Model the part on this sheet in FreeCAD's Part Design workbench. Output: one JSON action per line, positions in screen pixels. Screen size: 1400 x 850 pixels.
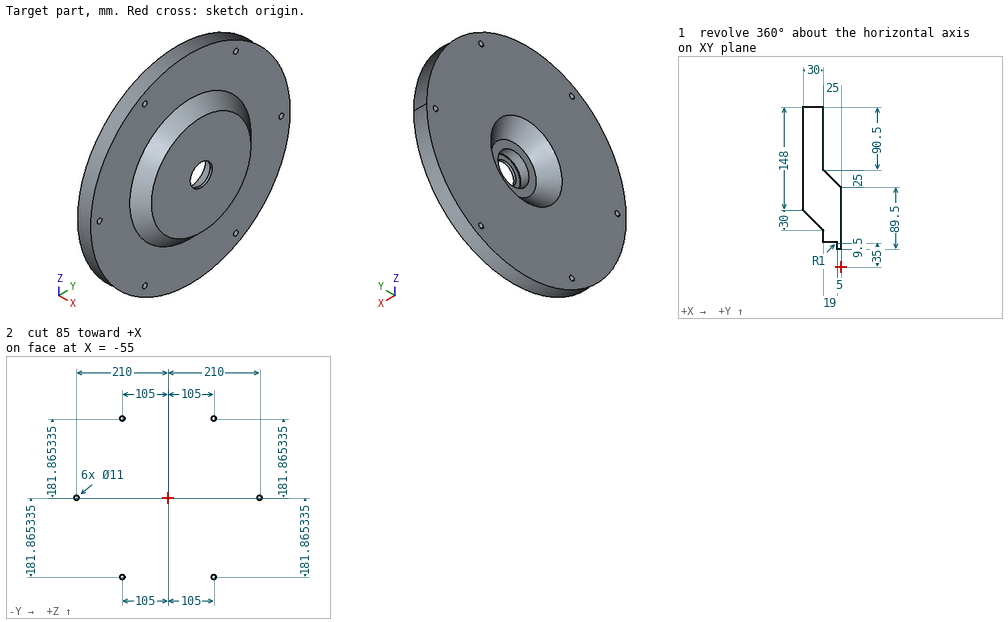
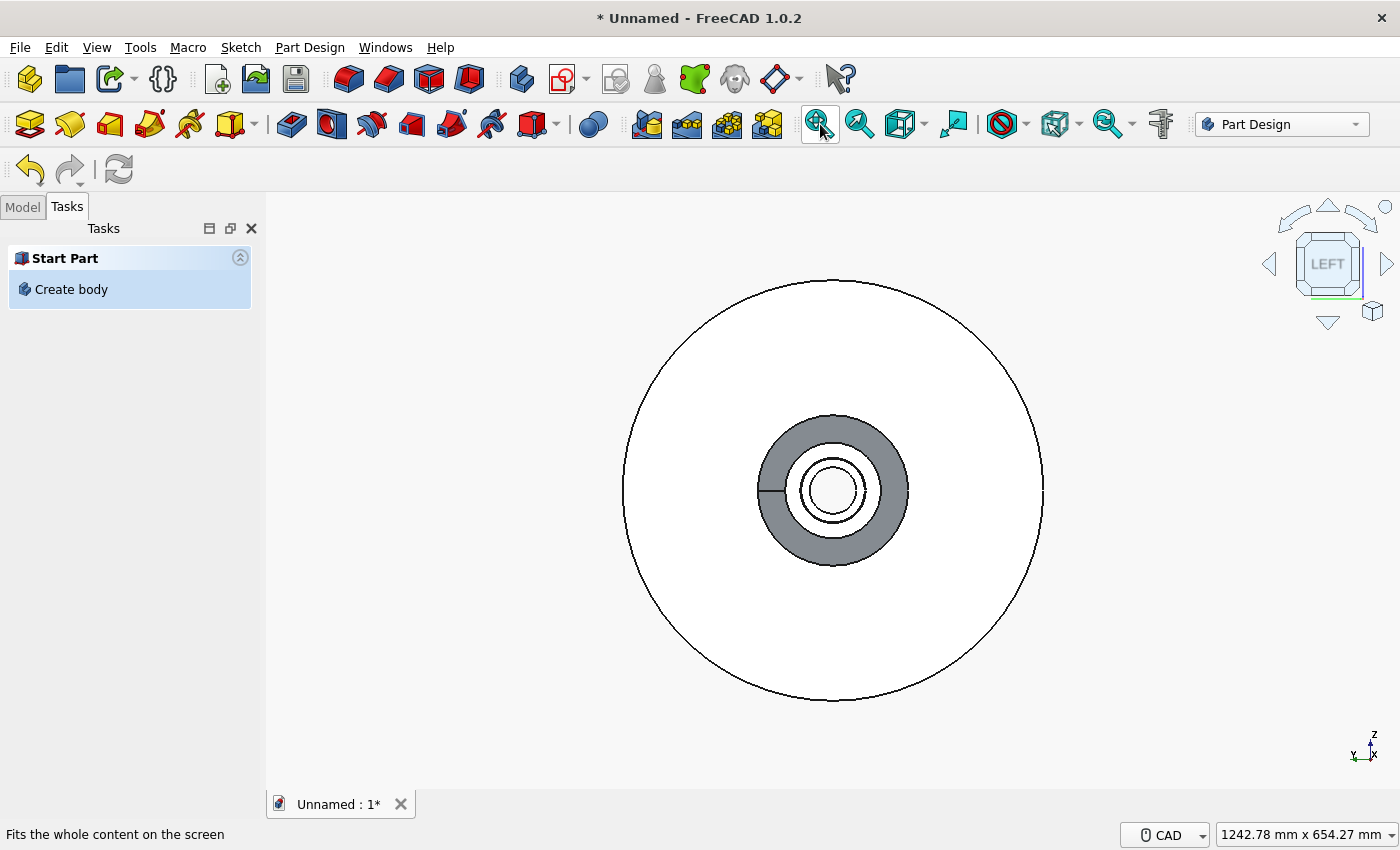
{"action": "left_click", "coordinate": [713, 550]}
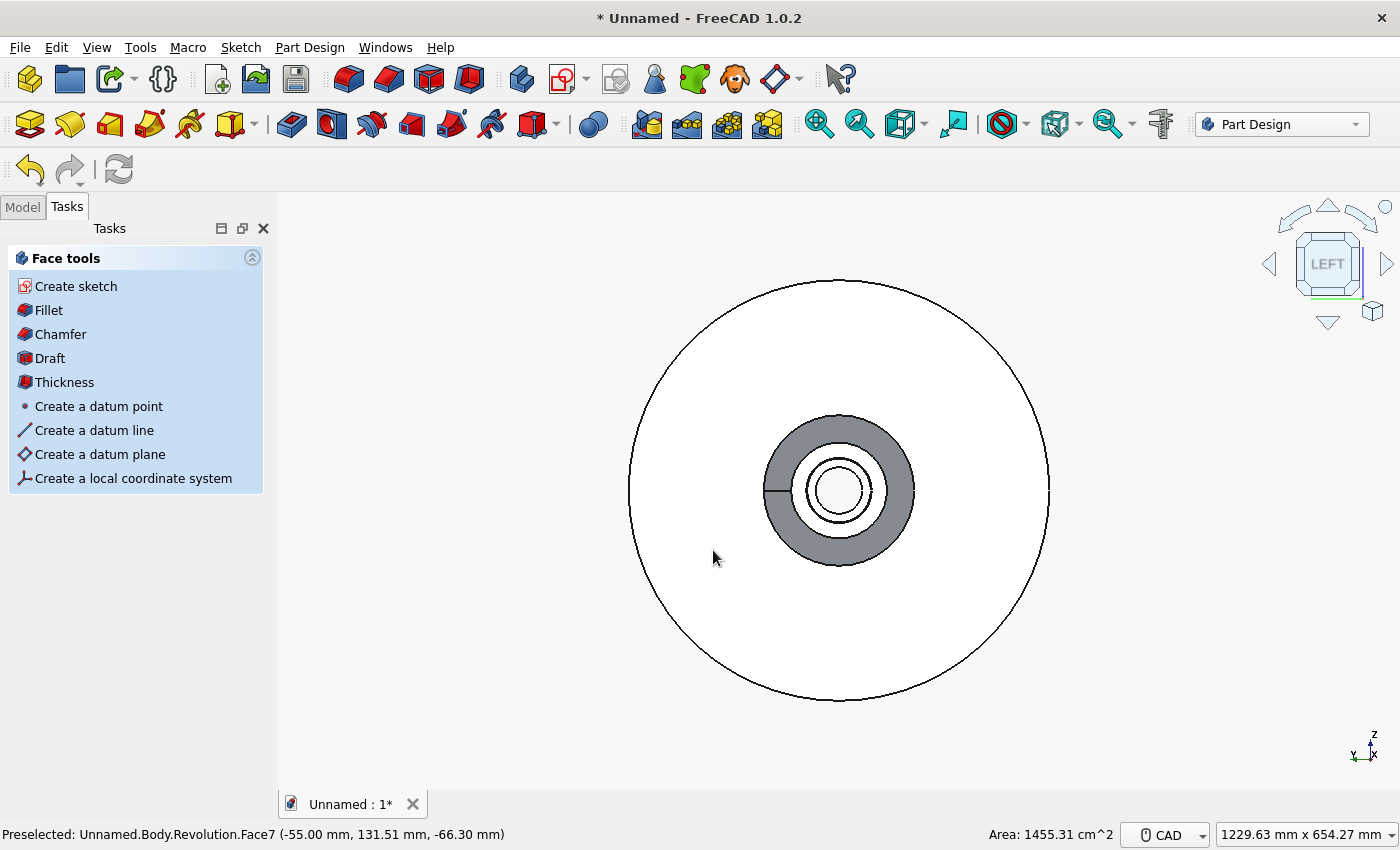
{"action": "left_click", "coordinate": [562, 80]}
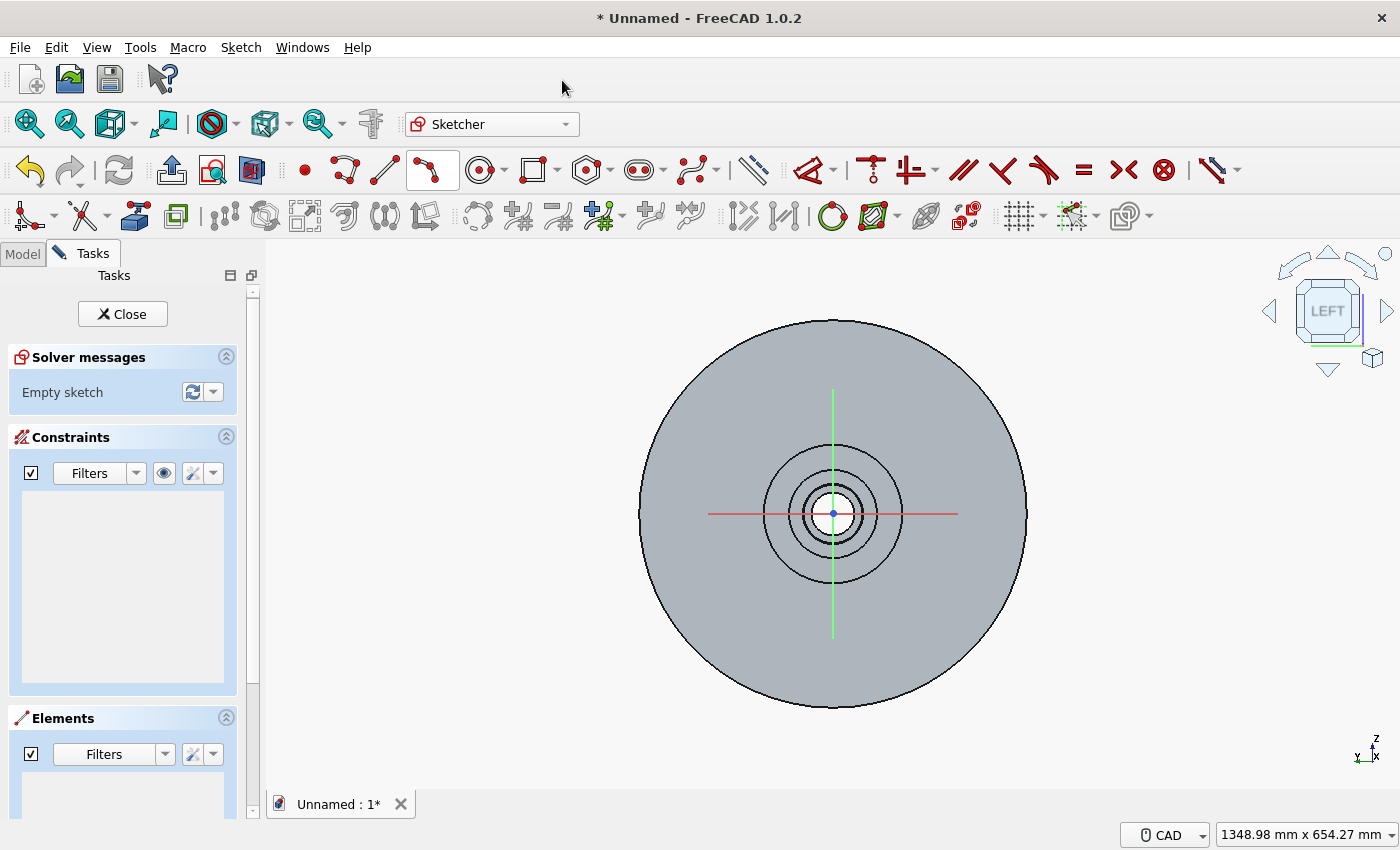
{"action": "left_click", "coordinate": [480, 170]}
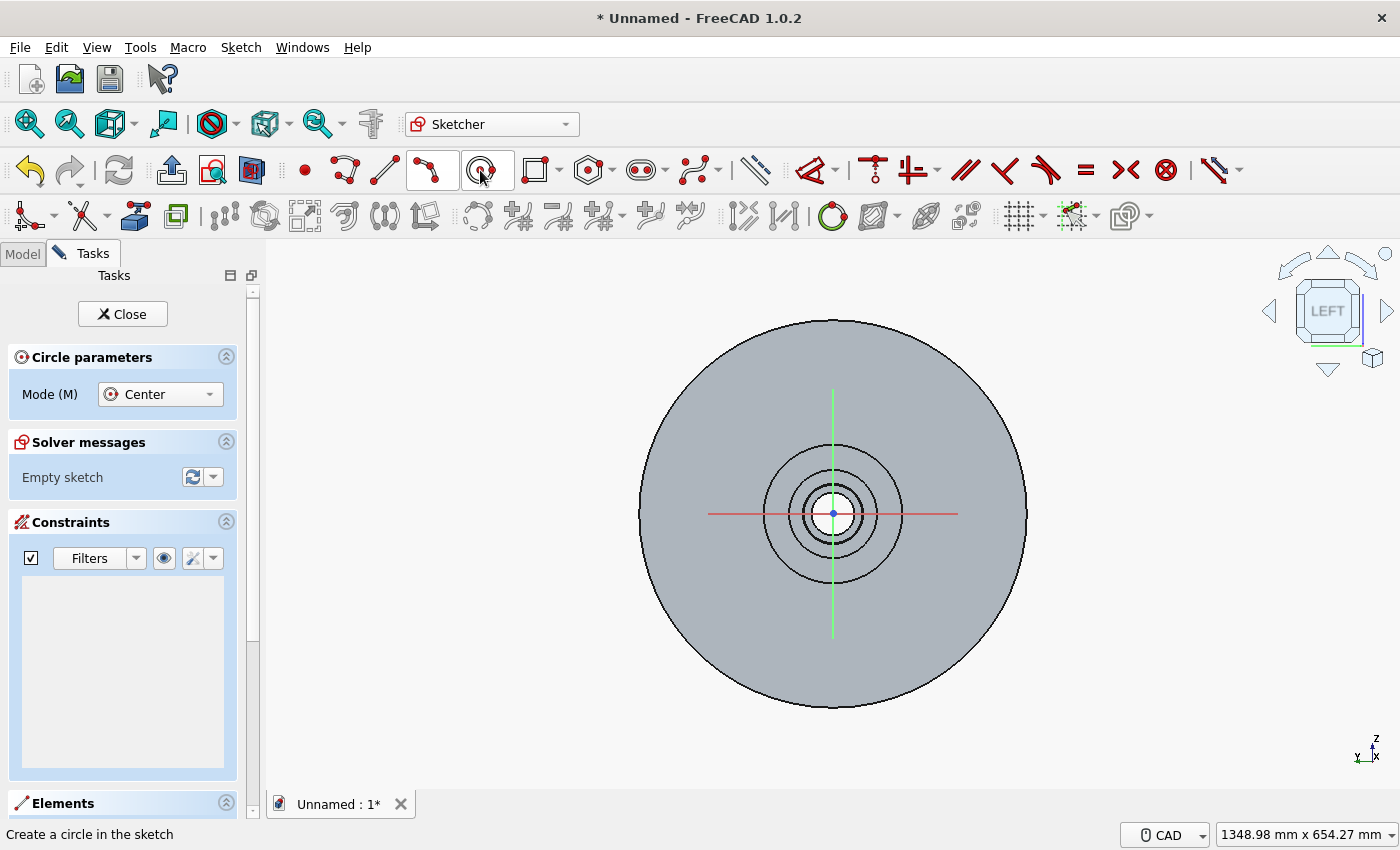
{"action": "scroll", "coordinate": [656, 514], "scroll_direction": "up", "scroll_amount": 8}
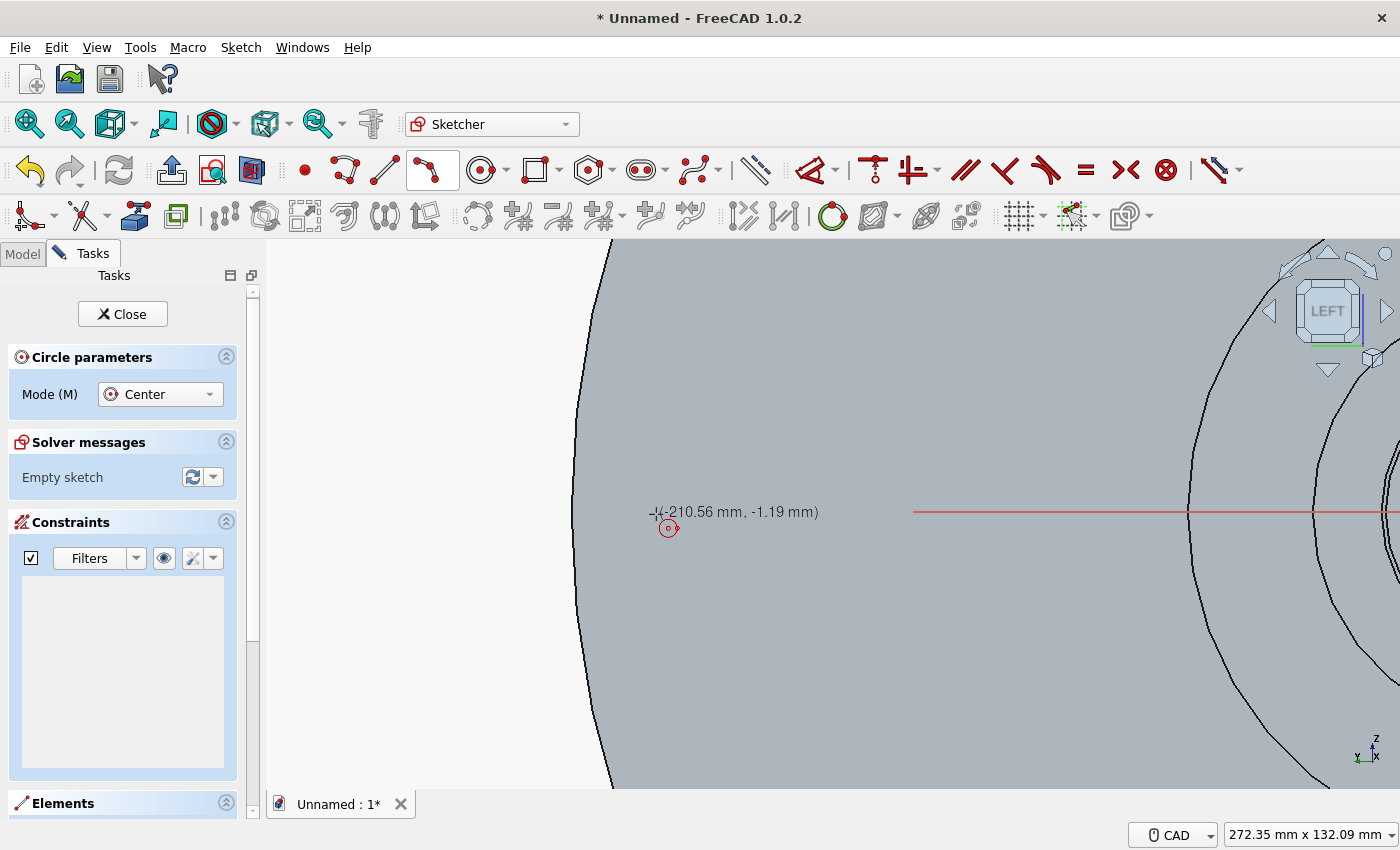
{"action": "scroll", "coordinate": [514, 515], "scroll_direction": "down", "scroll_amount": 7}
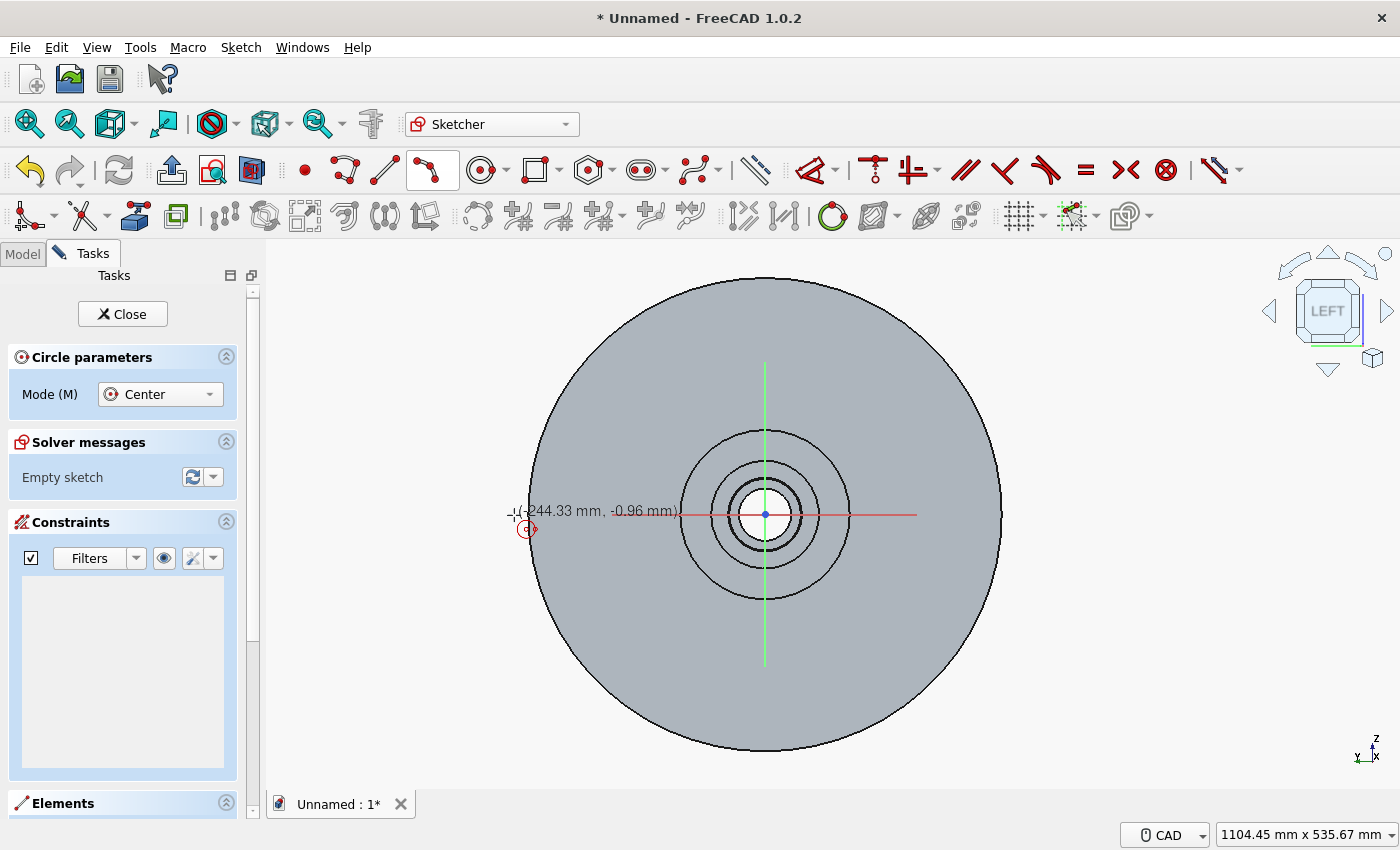
{"action": "left_click", "coordinate": [549, 515]}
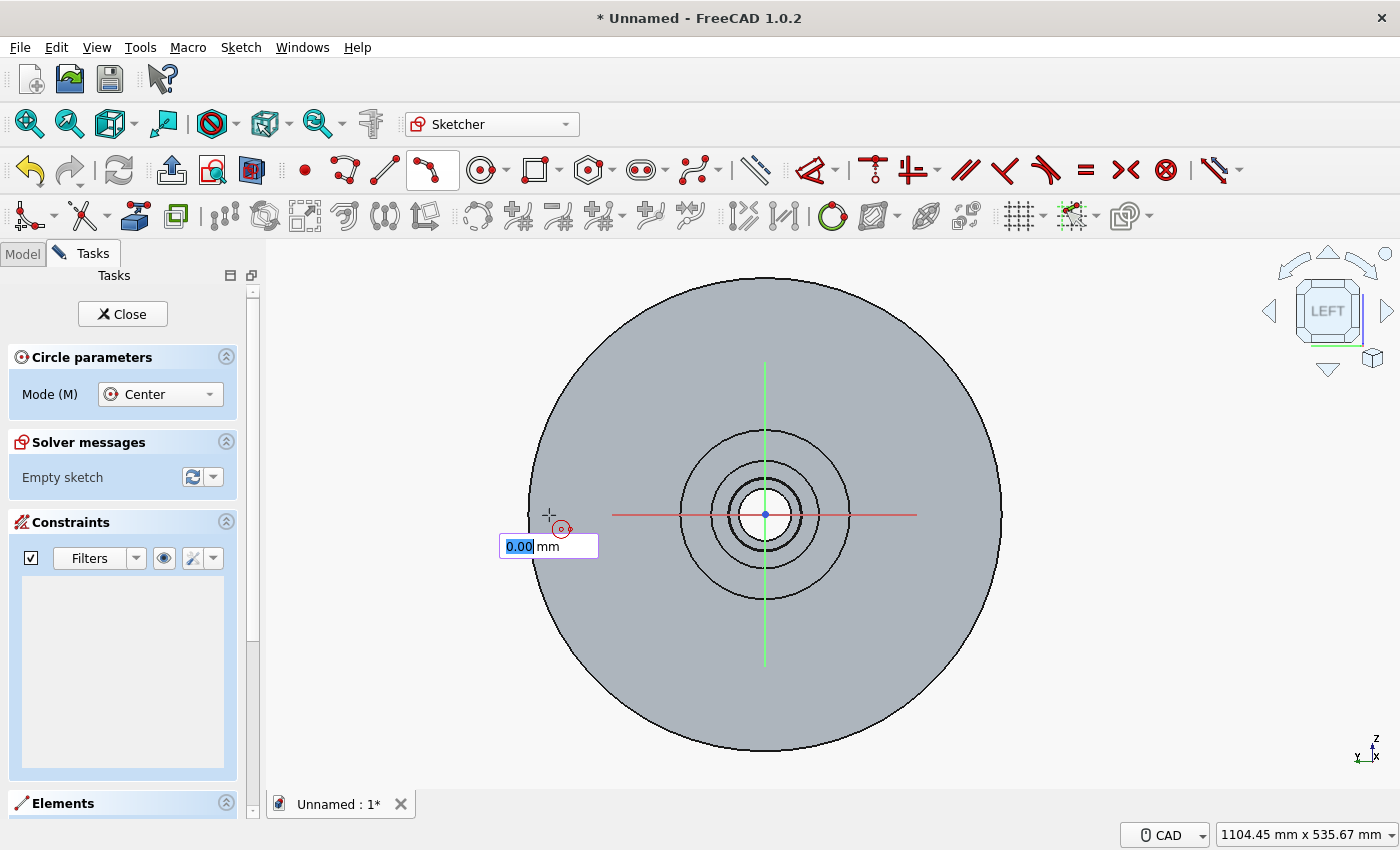
{"action": "scroll", "coordinate": [551, 509], "scroll_direction": "up", "scroll_amount": 6}
{"action": "mouse_move", "coordinate": [552, 509]}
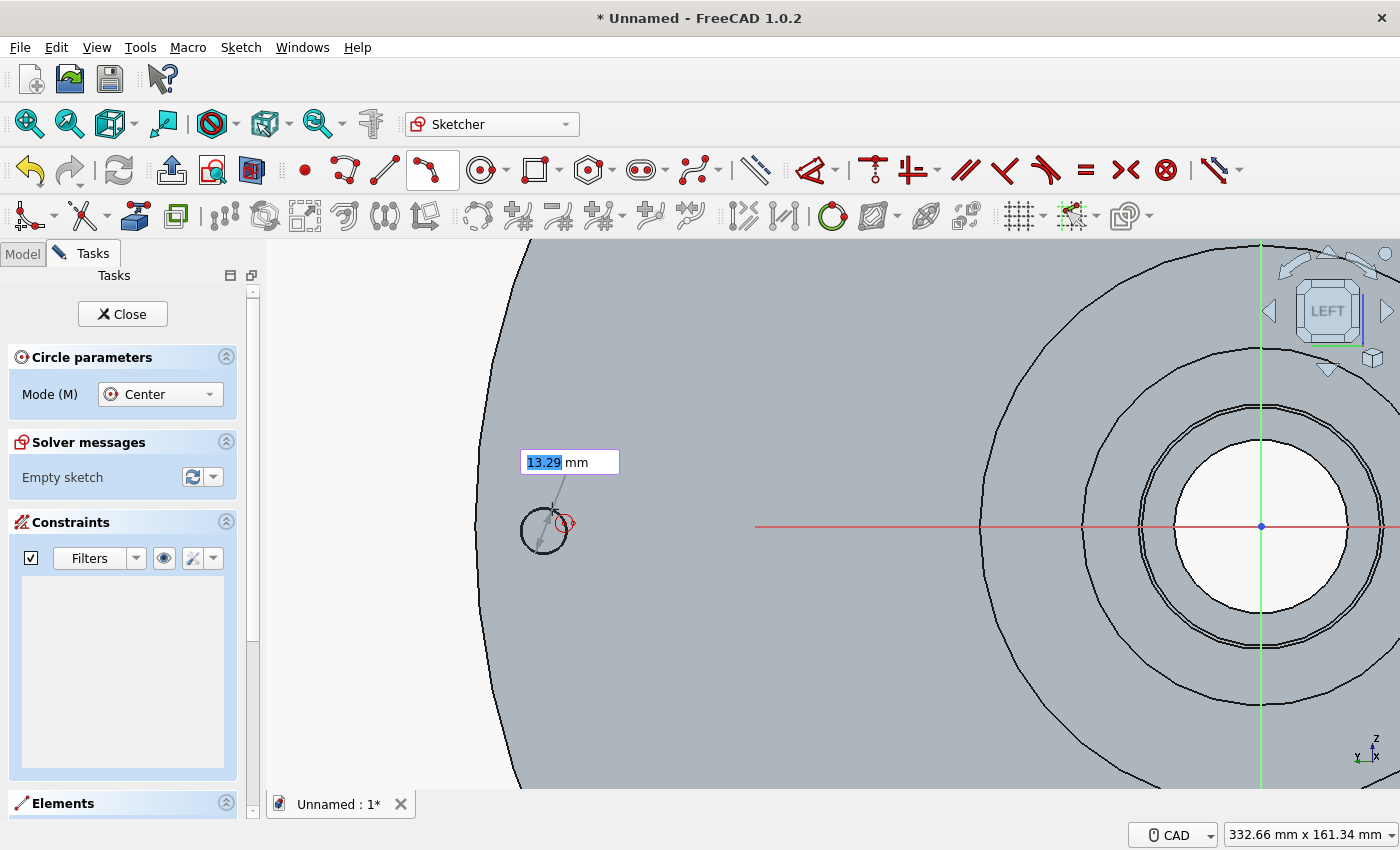
{"action": "type", "text": "11"}
{"action": "key", "text": "Return"}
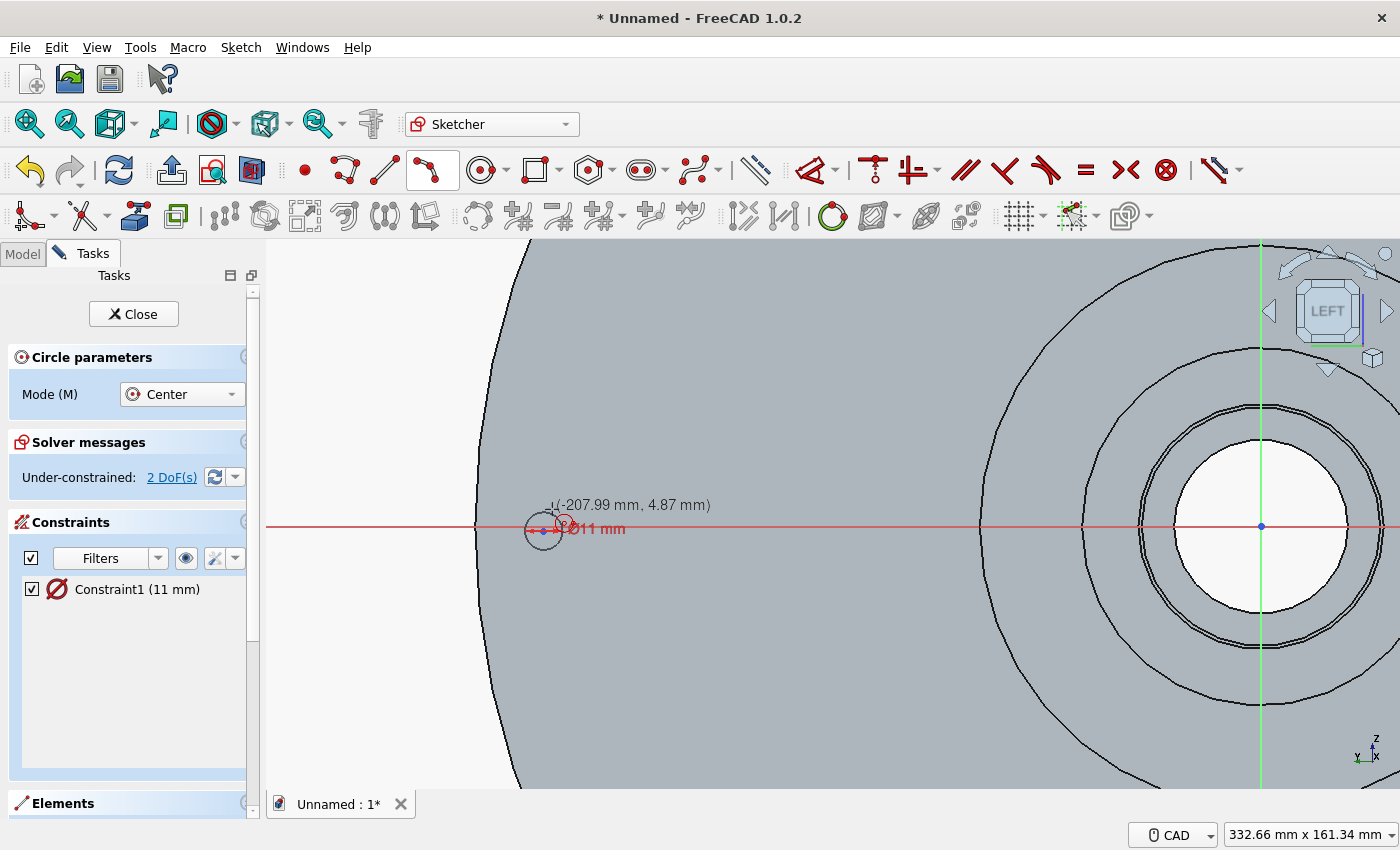
{"action": "scroll", "coordinate": [550, 509], "scroll_direction": "down", "scroll_amount": 6}